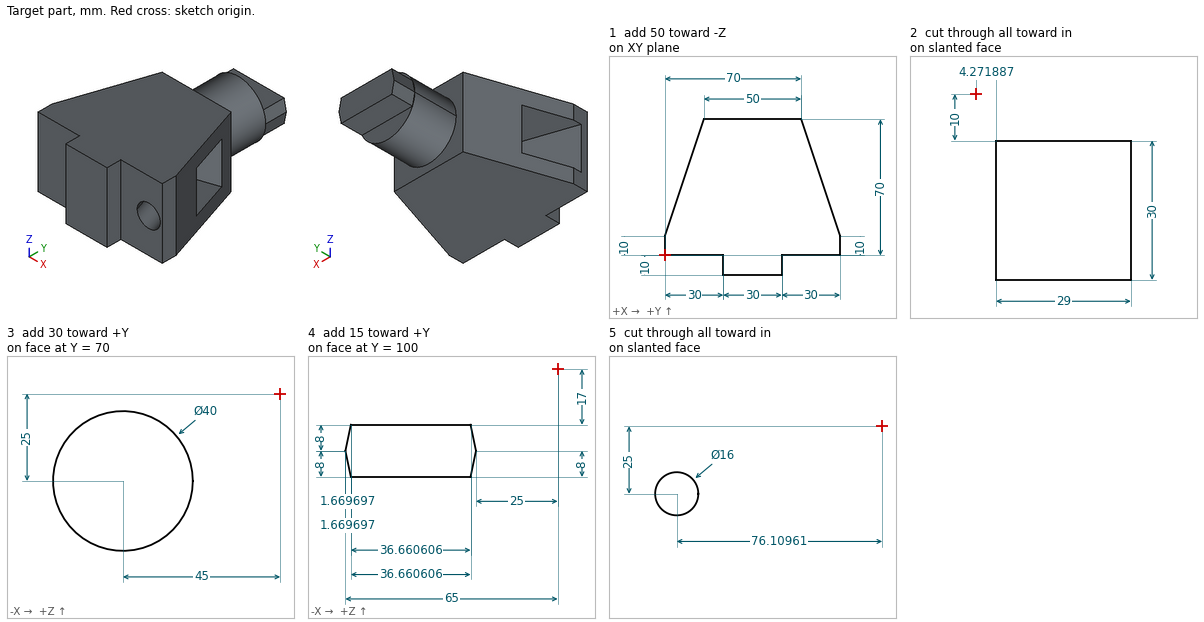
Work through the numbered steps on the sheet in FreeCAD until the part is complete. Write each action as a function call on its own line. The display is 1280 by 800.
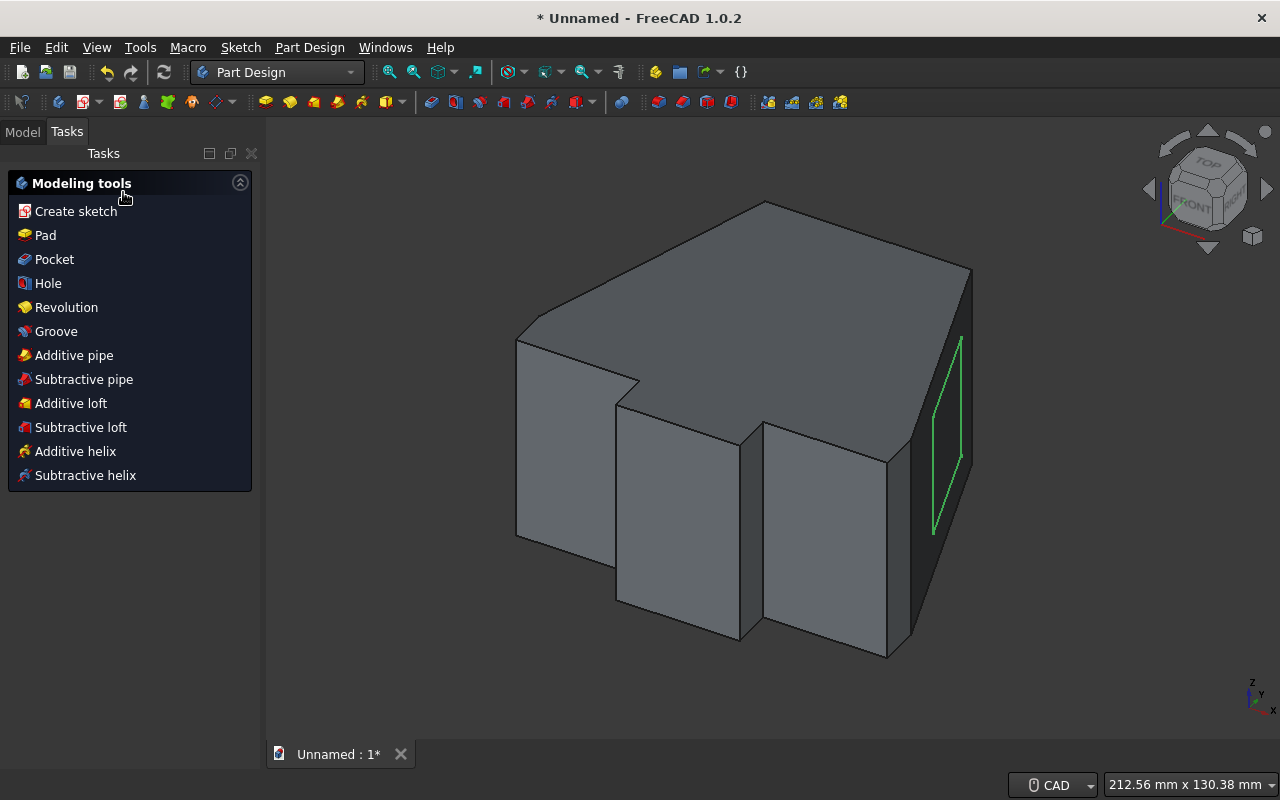
click(432, 102)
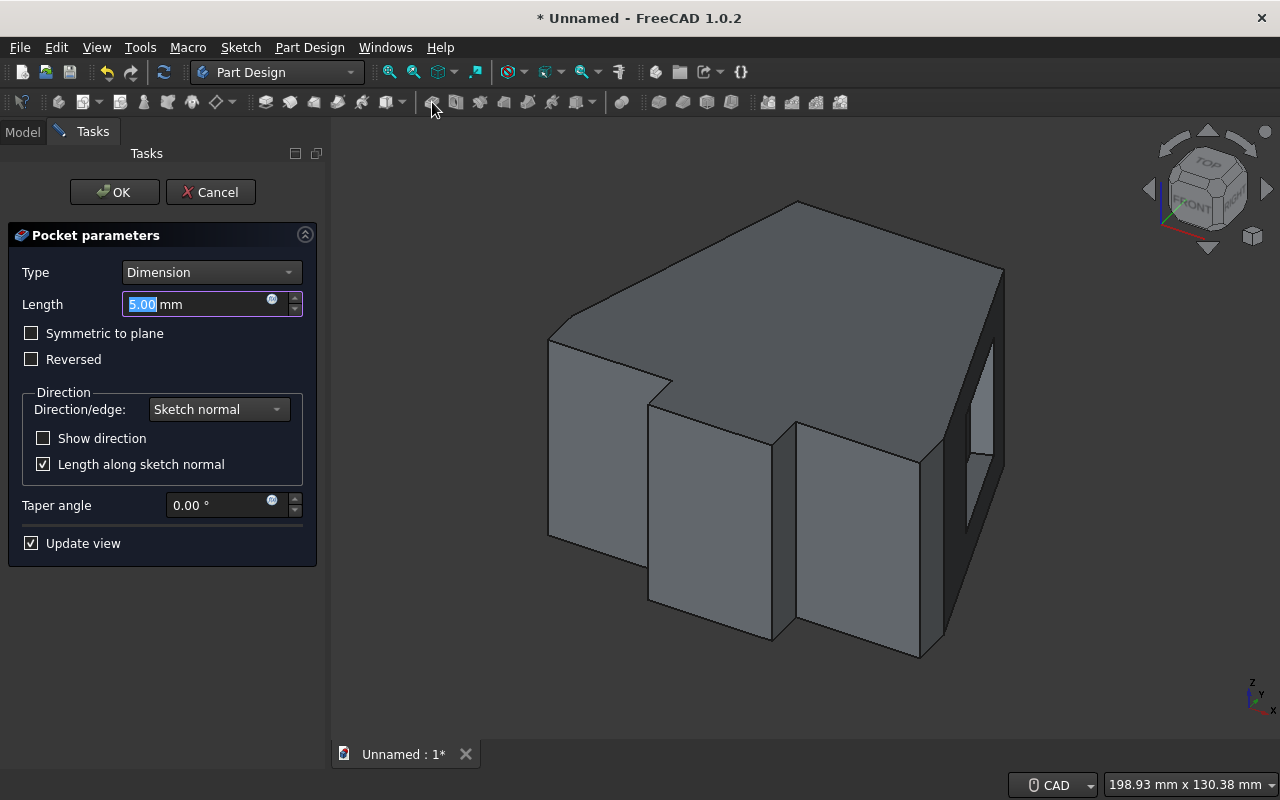
click(212, 272)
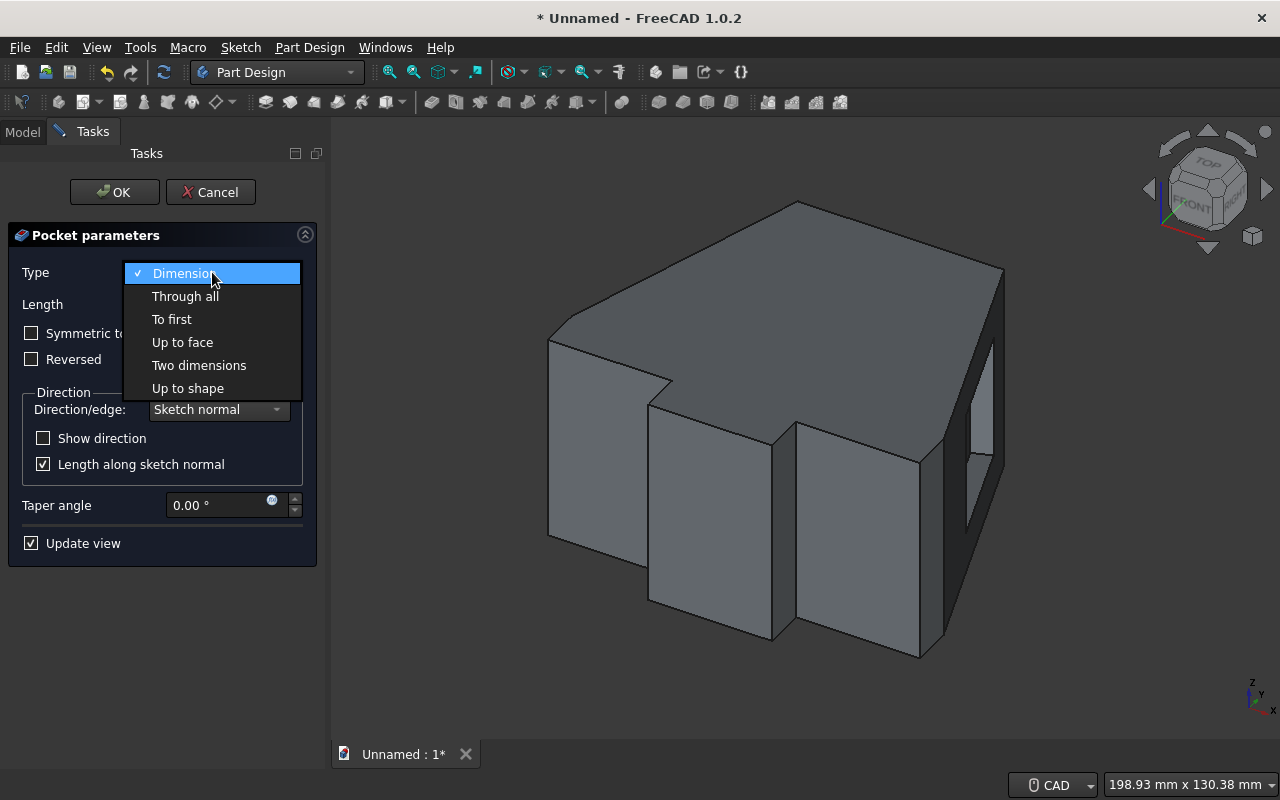
click(212, 296)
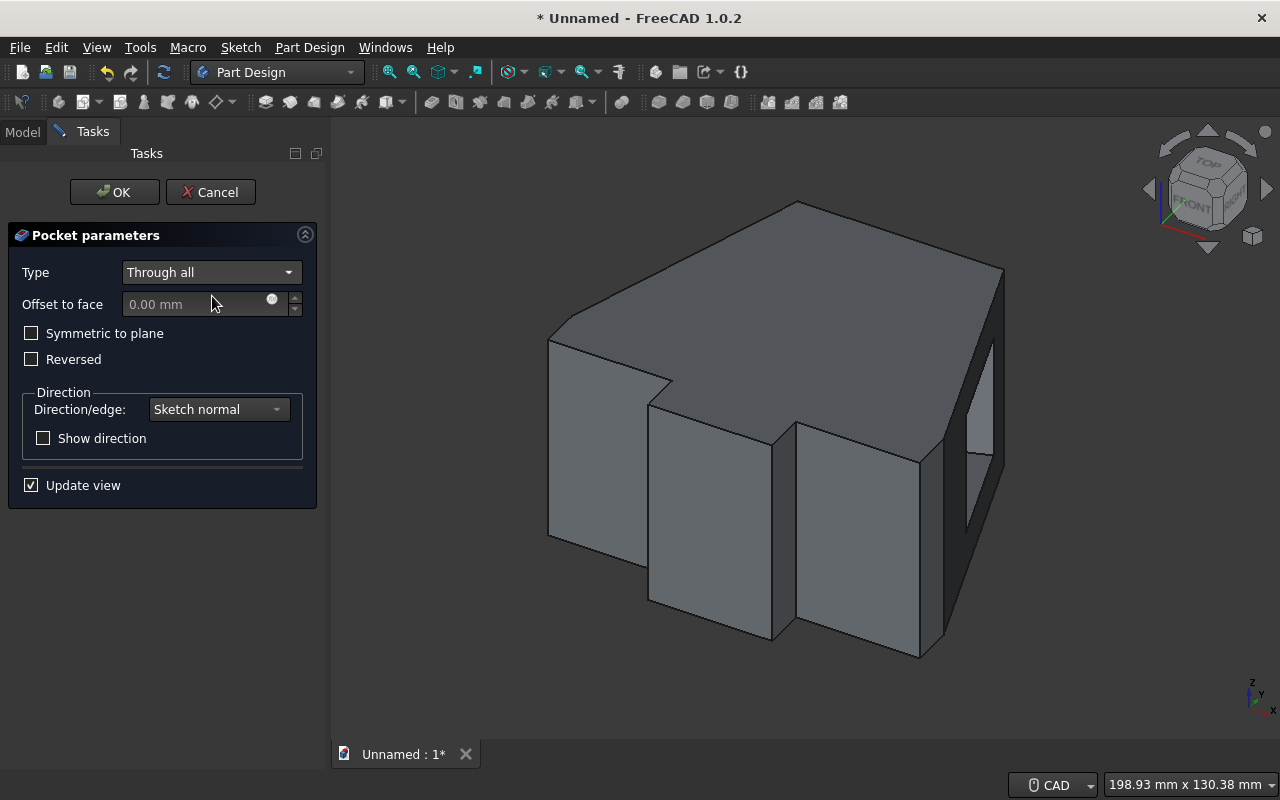
click(115, 192)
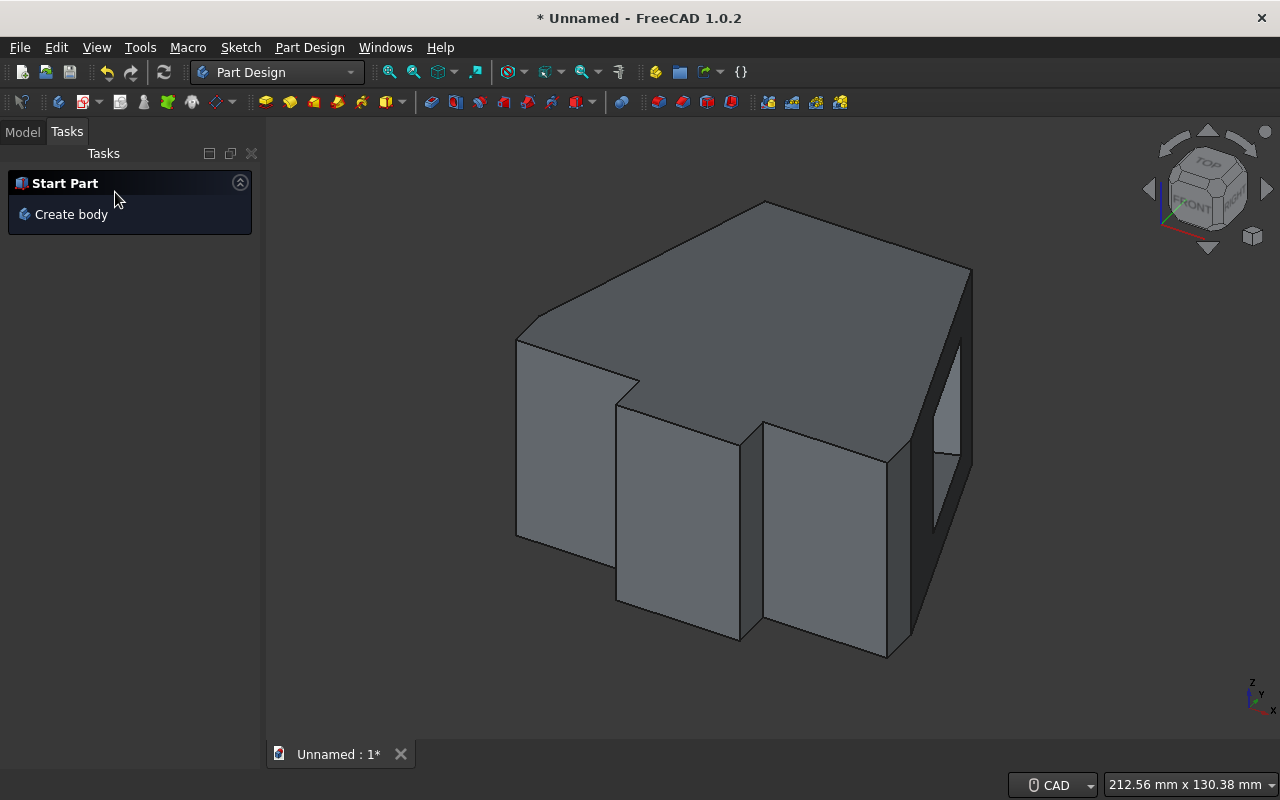
key(4)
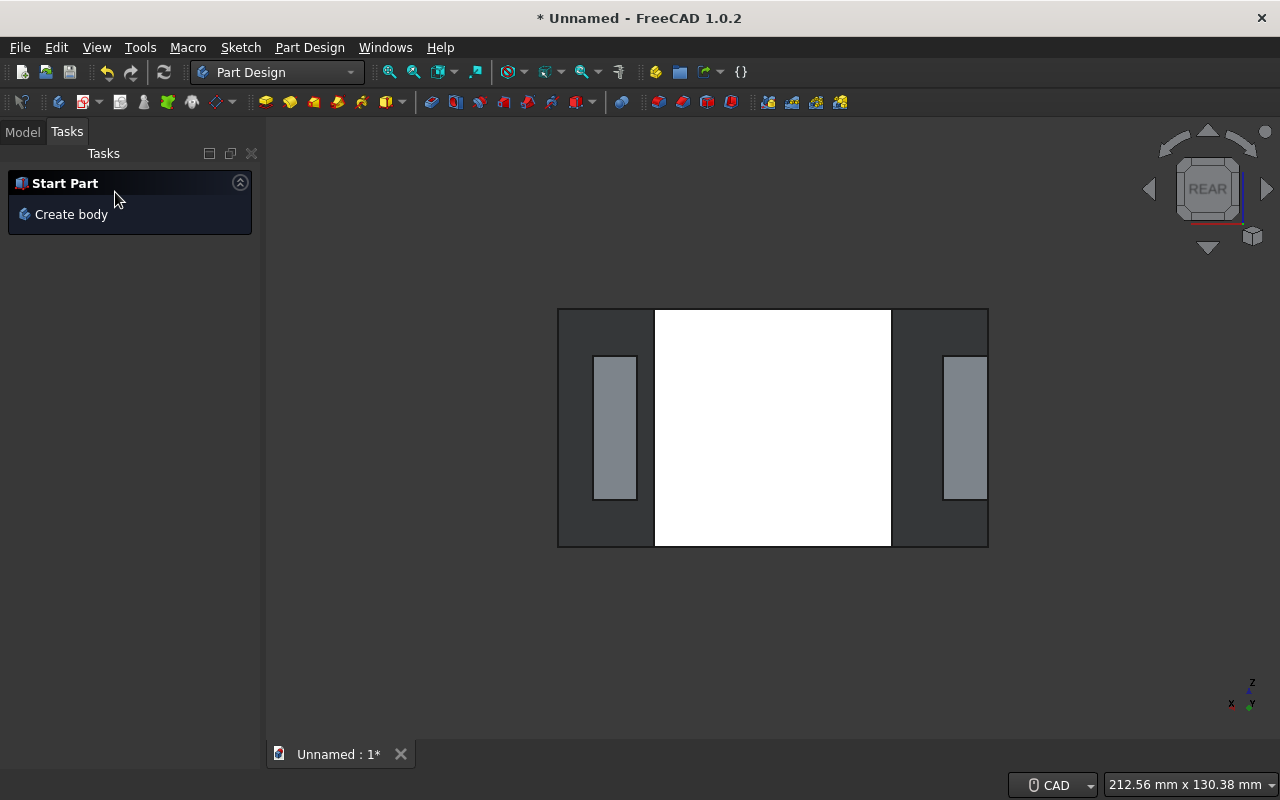
key(v)
key(f)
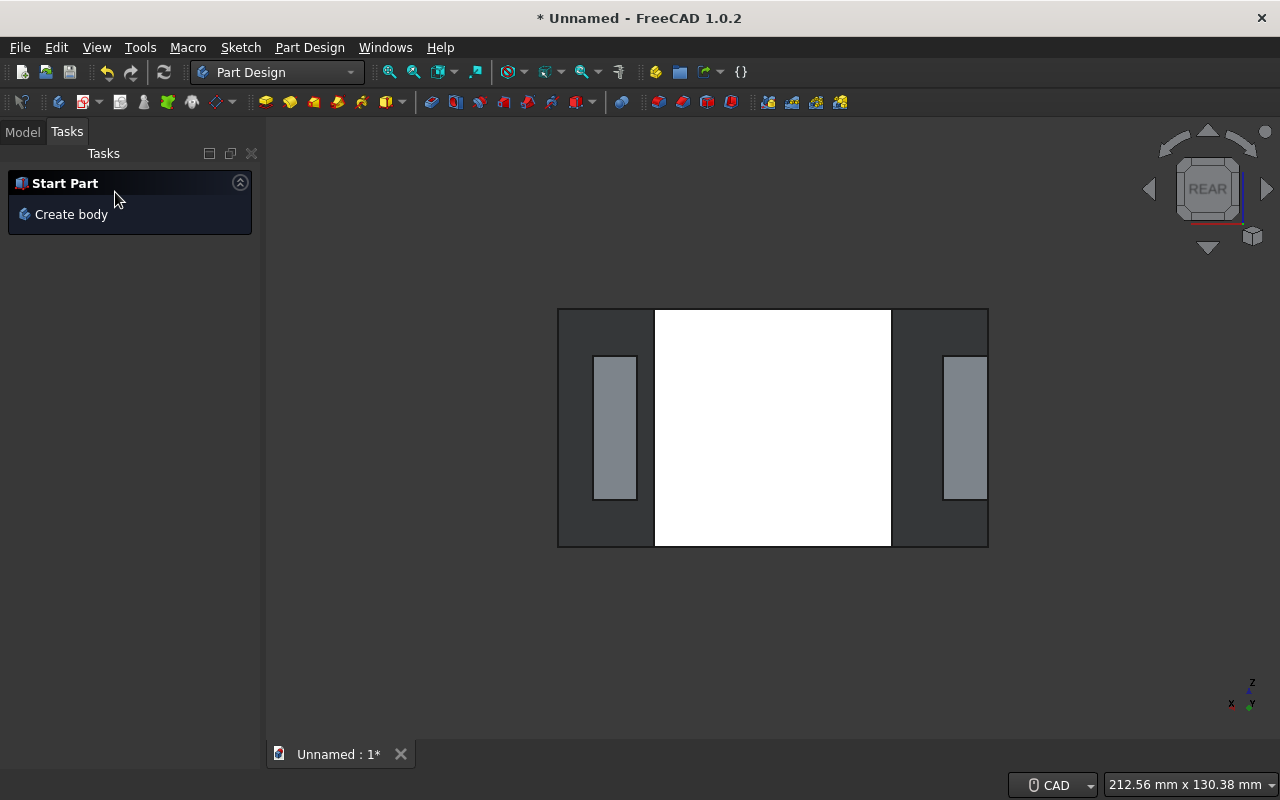
click(773, 427)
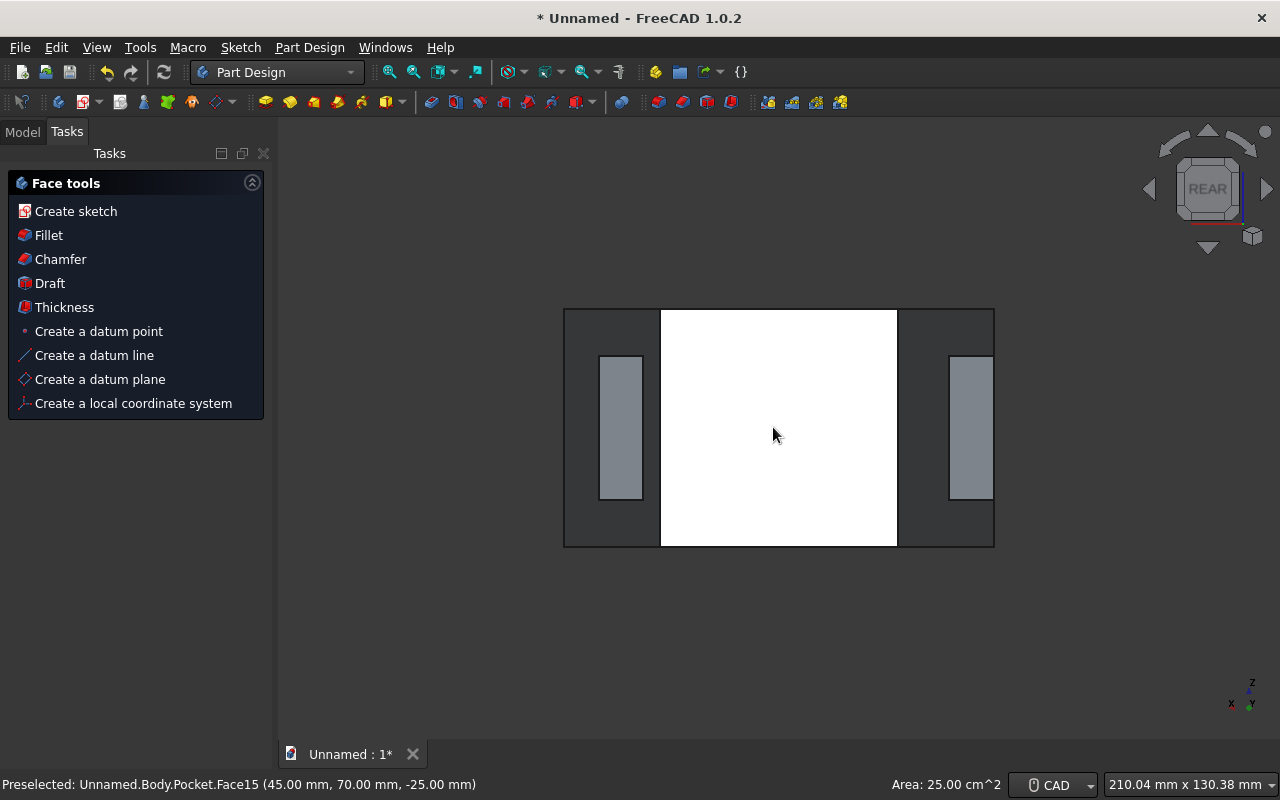
click(84, 102)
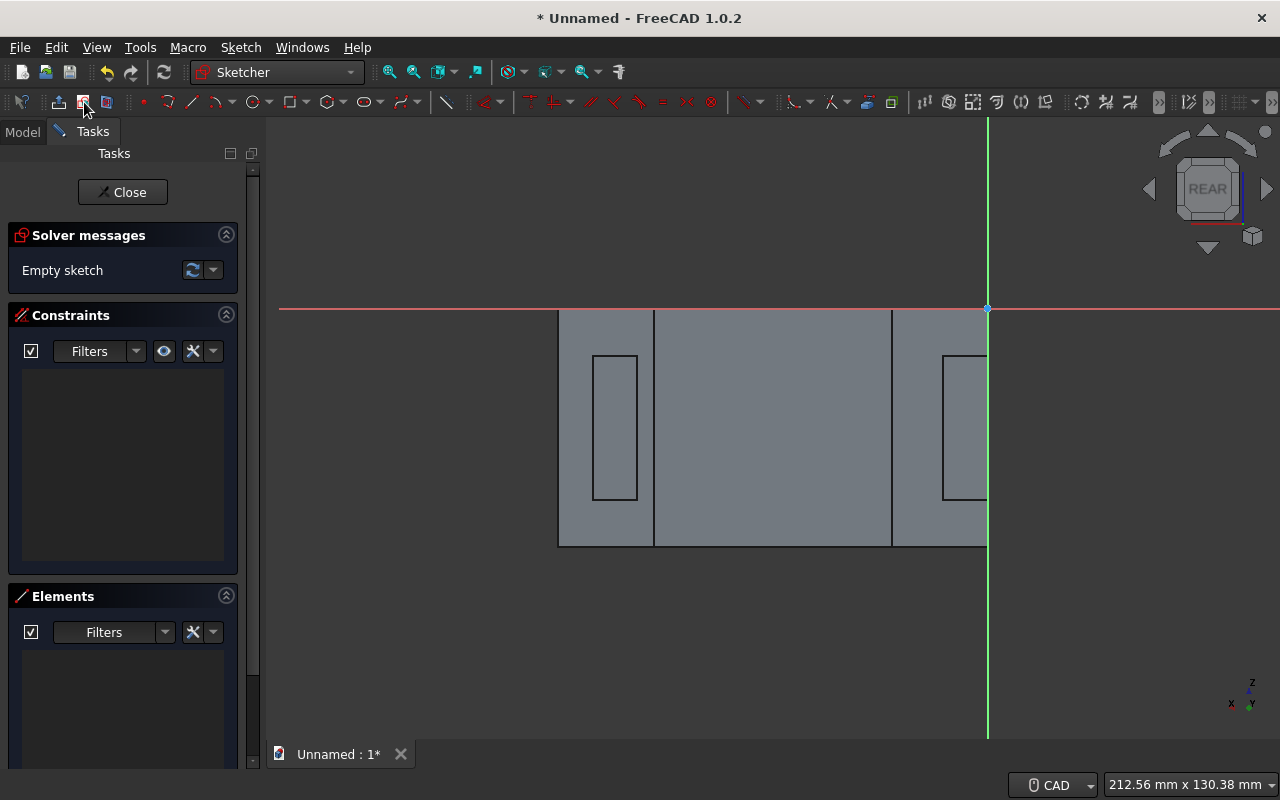
scroll(988, 402, up, 3)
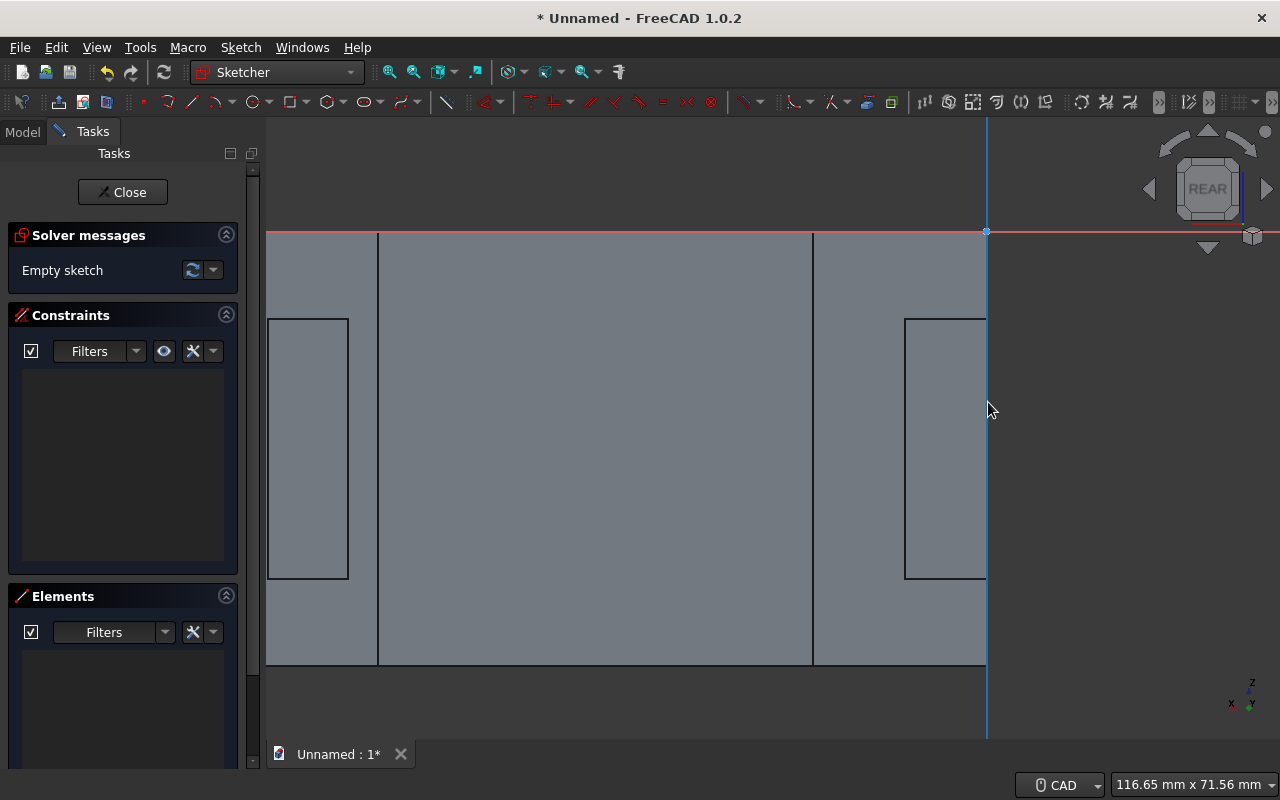
key(g)
key(c)